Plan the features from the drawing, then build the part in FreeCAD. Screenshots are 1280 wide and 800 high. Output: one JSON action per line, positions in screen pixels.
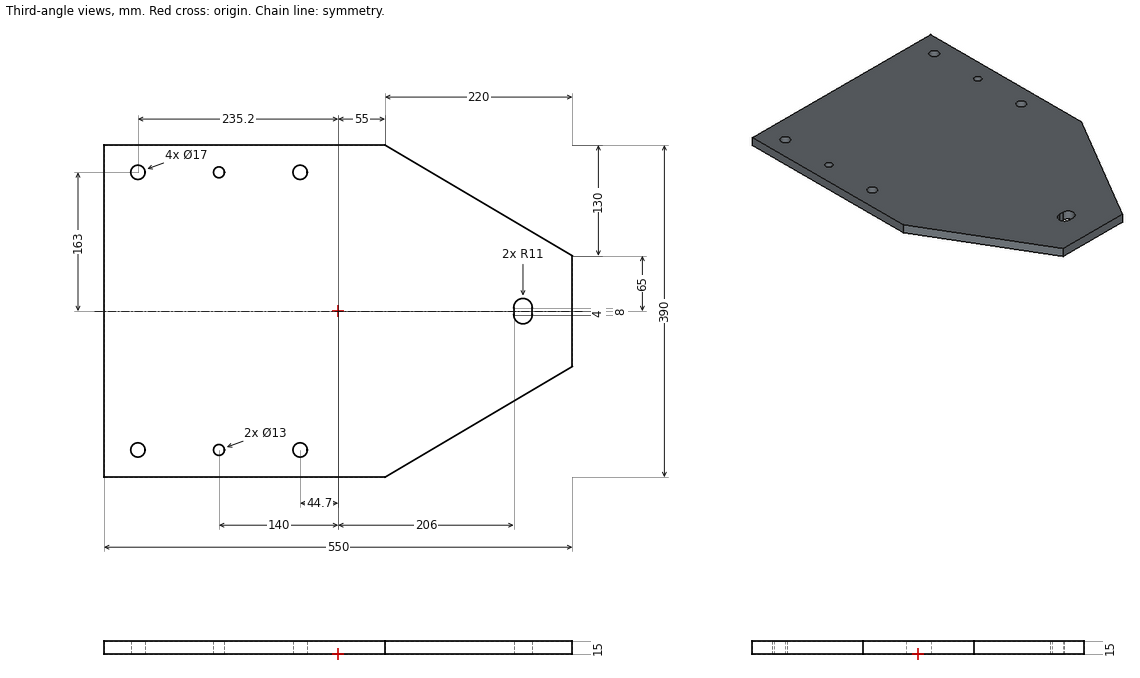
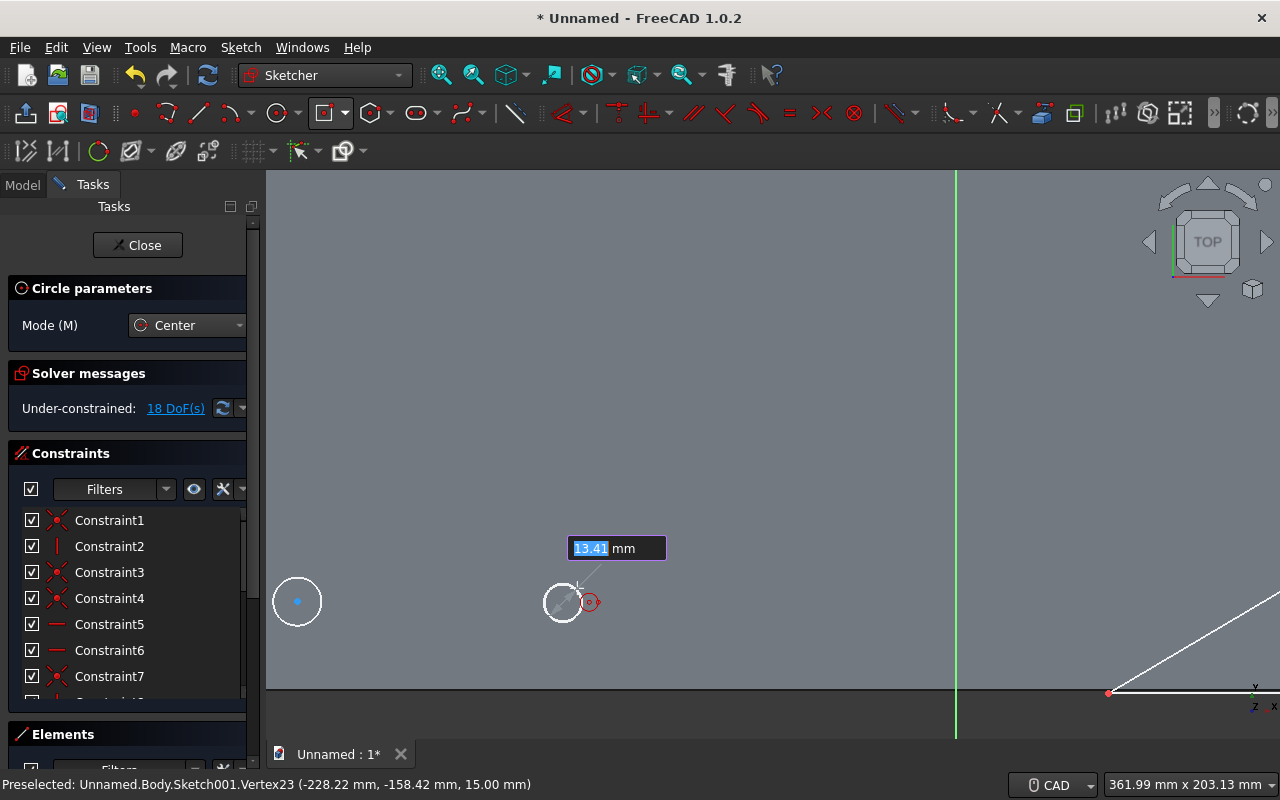
{"action": "left_click", "coordinate": [577, 587]}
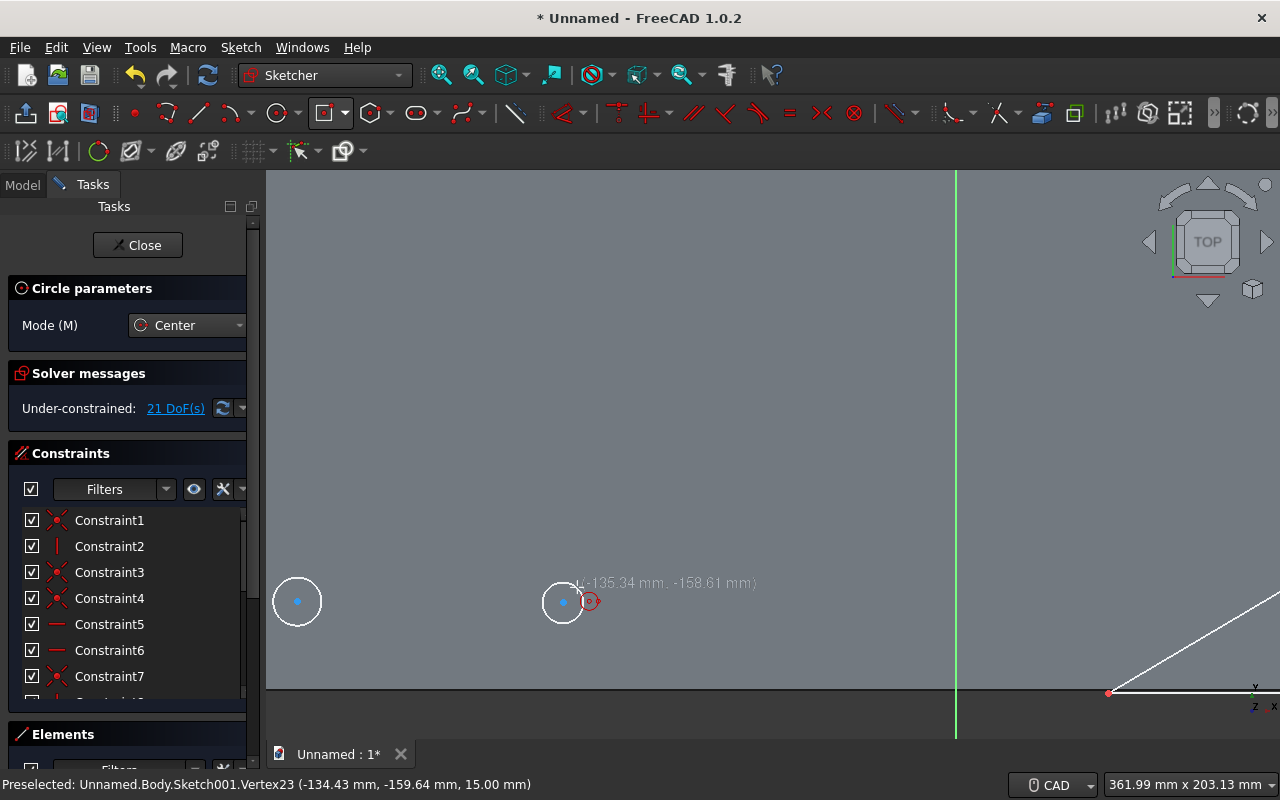
{"action": "left_click", "coordinate": [831, 600]}
{"action": "left_click", "coordinate": [848, 583]}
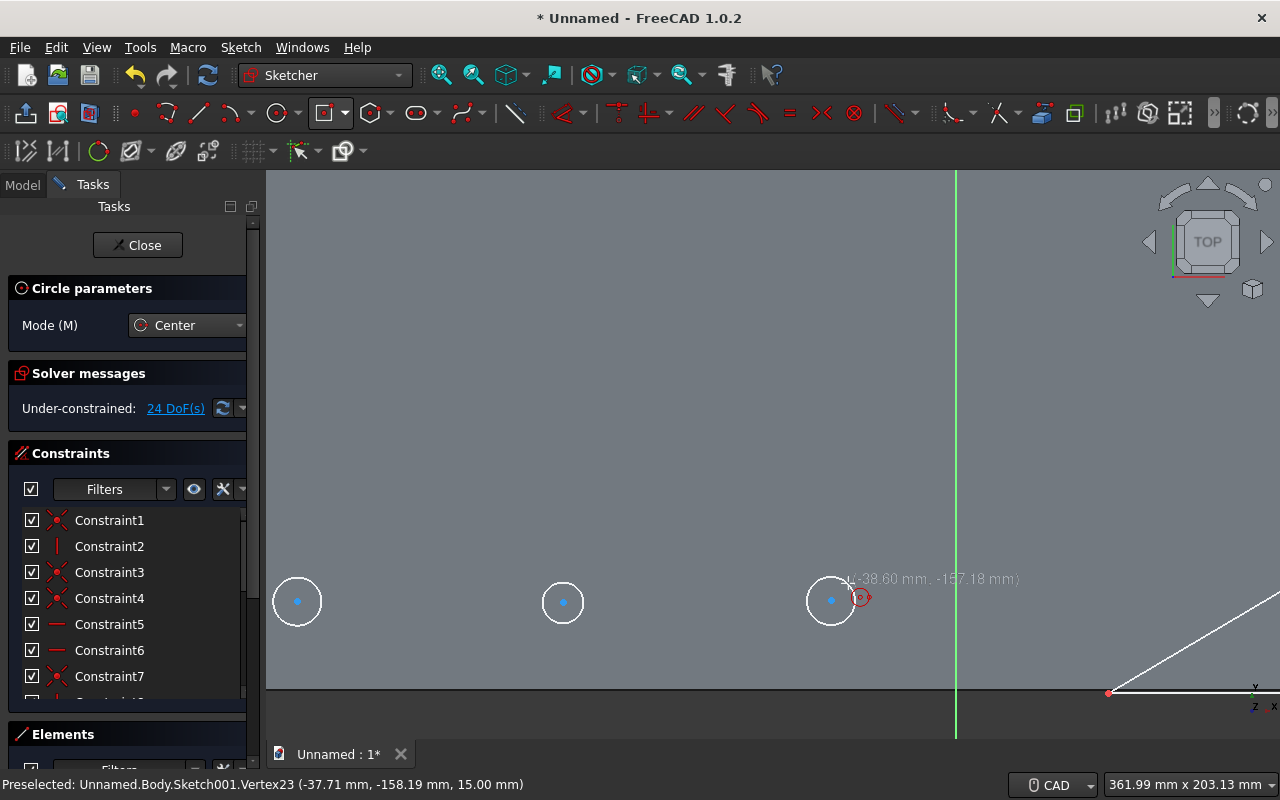
{"action": "scroll", "coordinate": [577, 588], "scroll_direction": "down", "scroll_amount": 6}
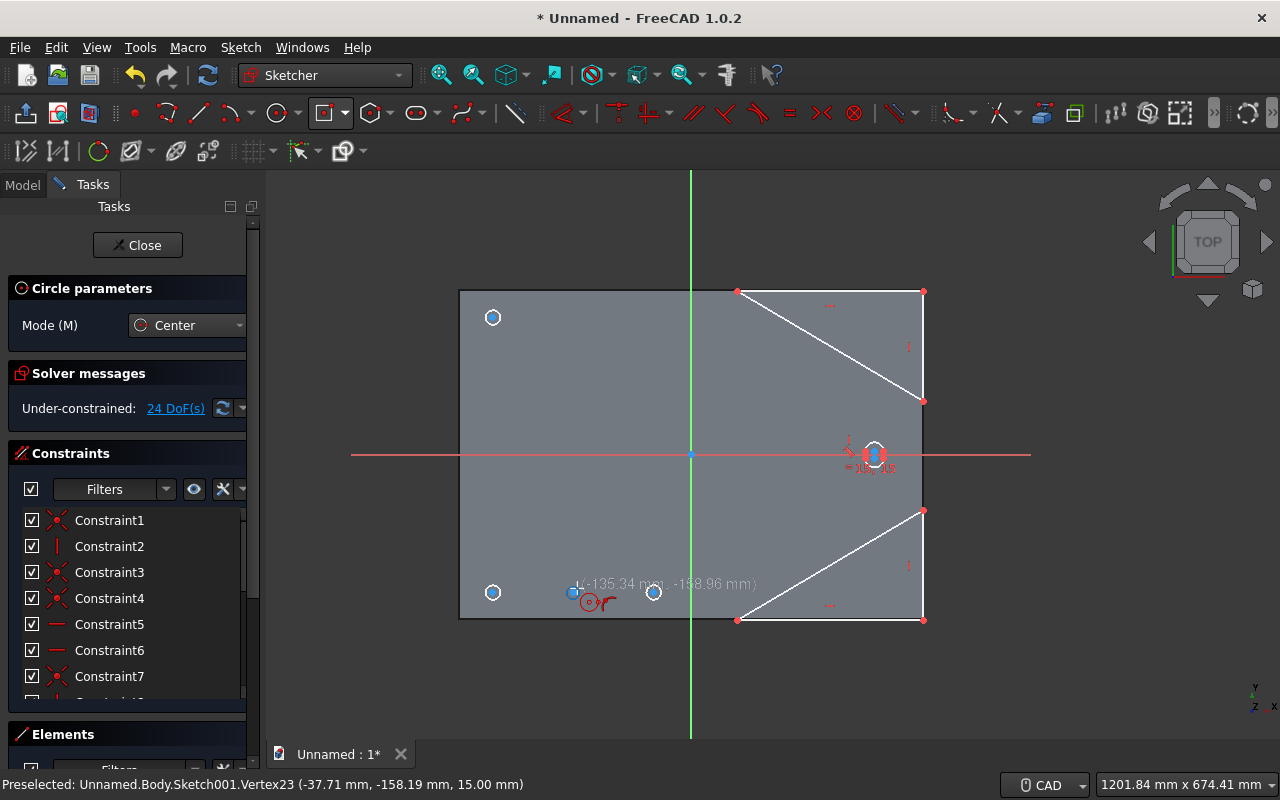
{"action": "scroll", "coordinate": [573, 317], "scroll_direction": "up", "scroll_amount": 8}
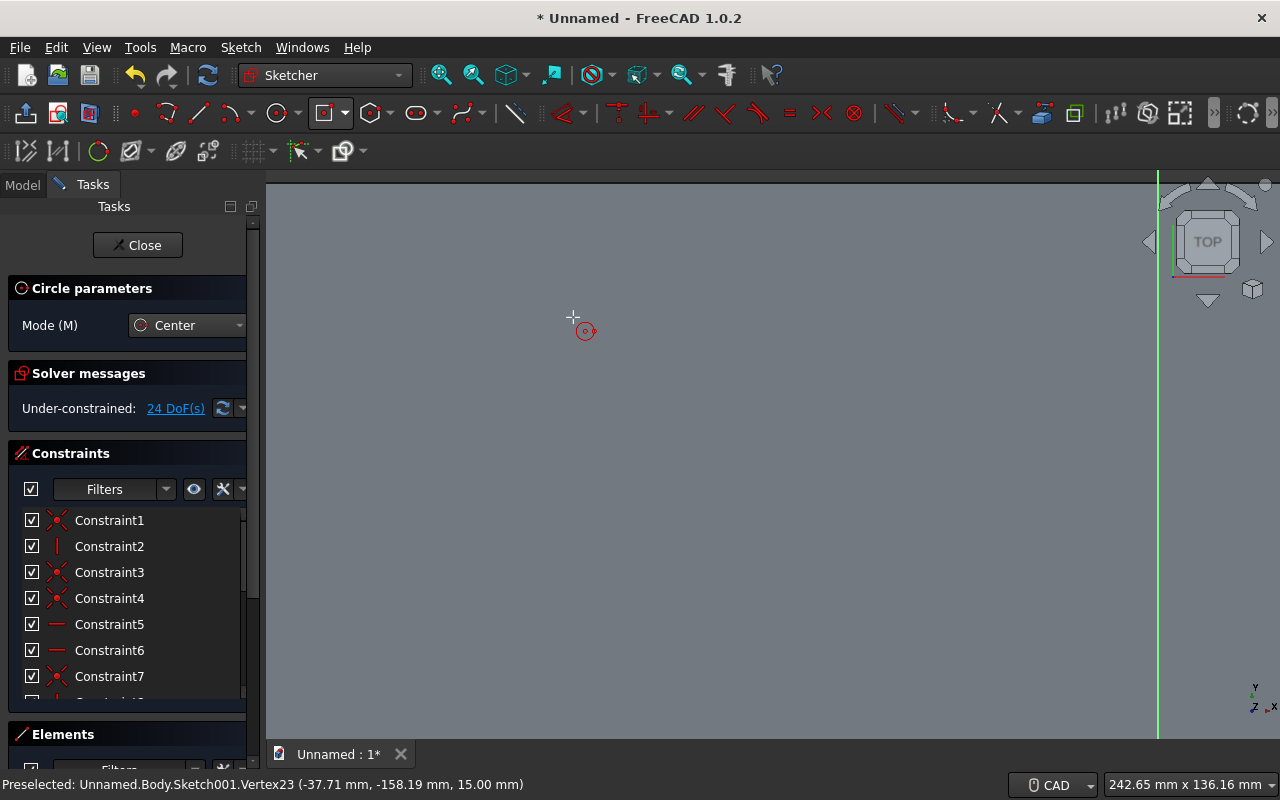
{"action": "scroll", "coordinate": [573, 317], "scroll_direction": "down", "scroll_amount": 8}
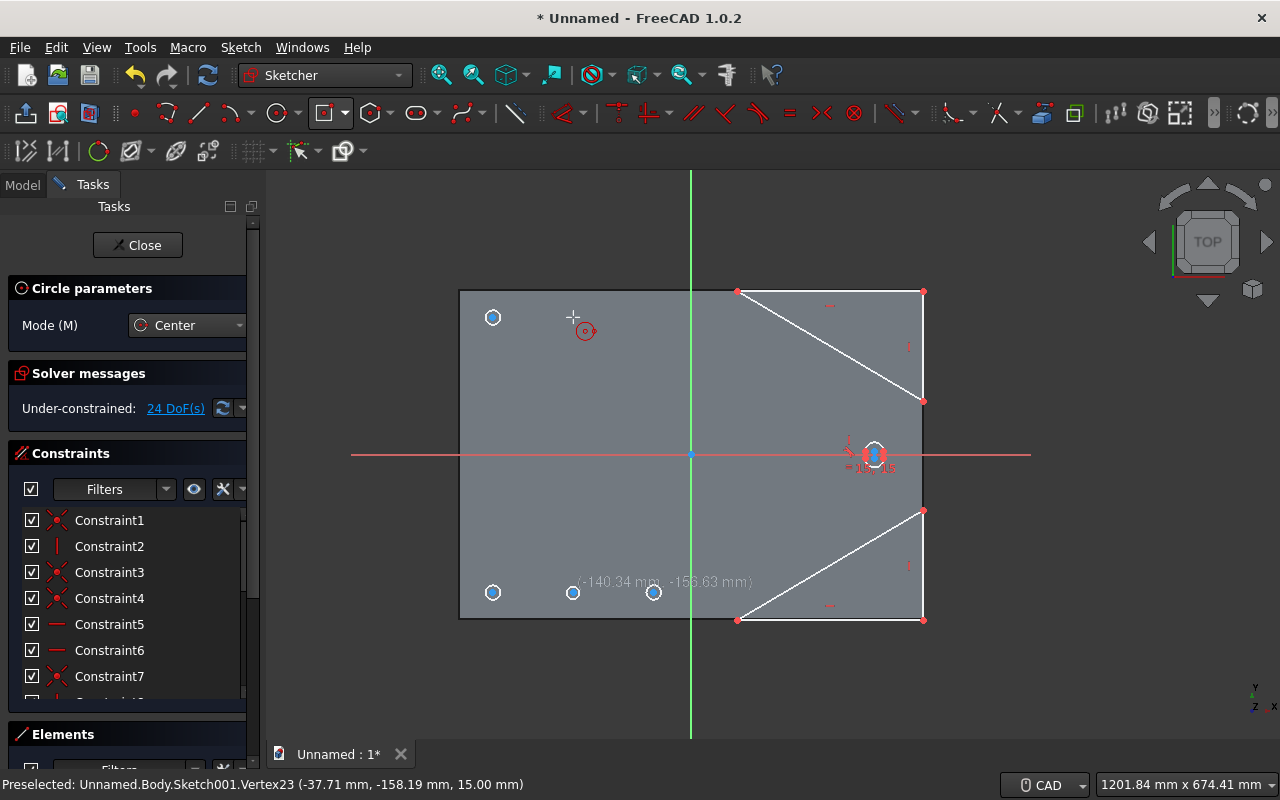
{"action": "left_click", "coordinate": [573, 317]}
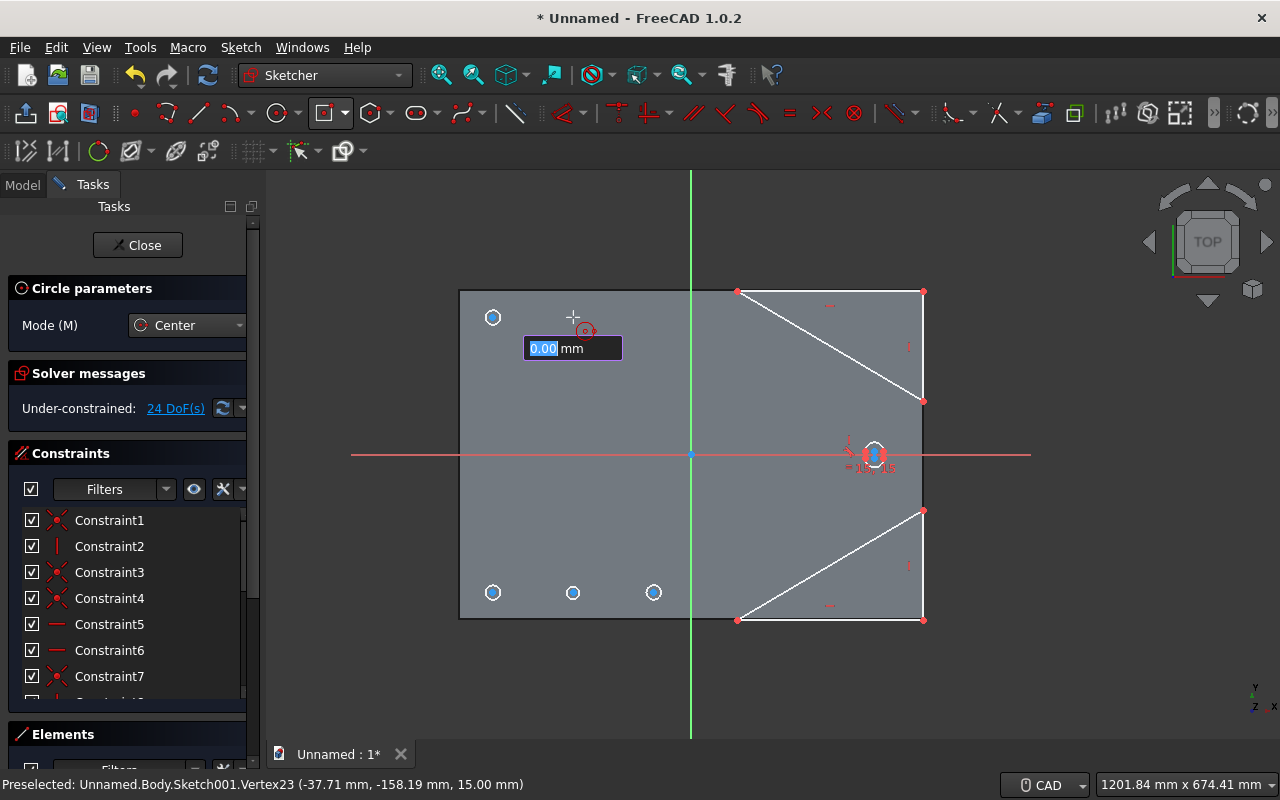
{"action": "scroll", "coordinate": [577, 313], "scroll_direction": "up", "scroll_amount": 6}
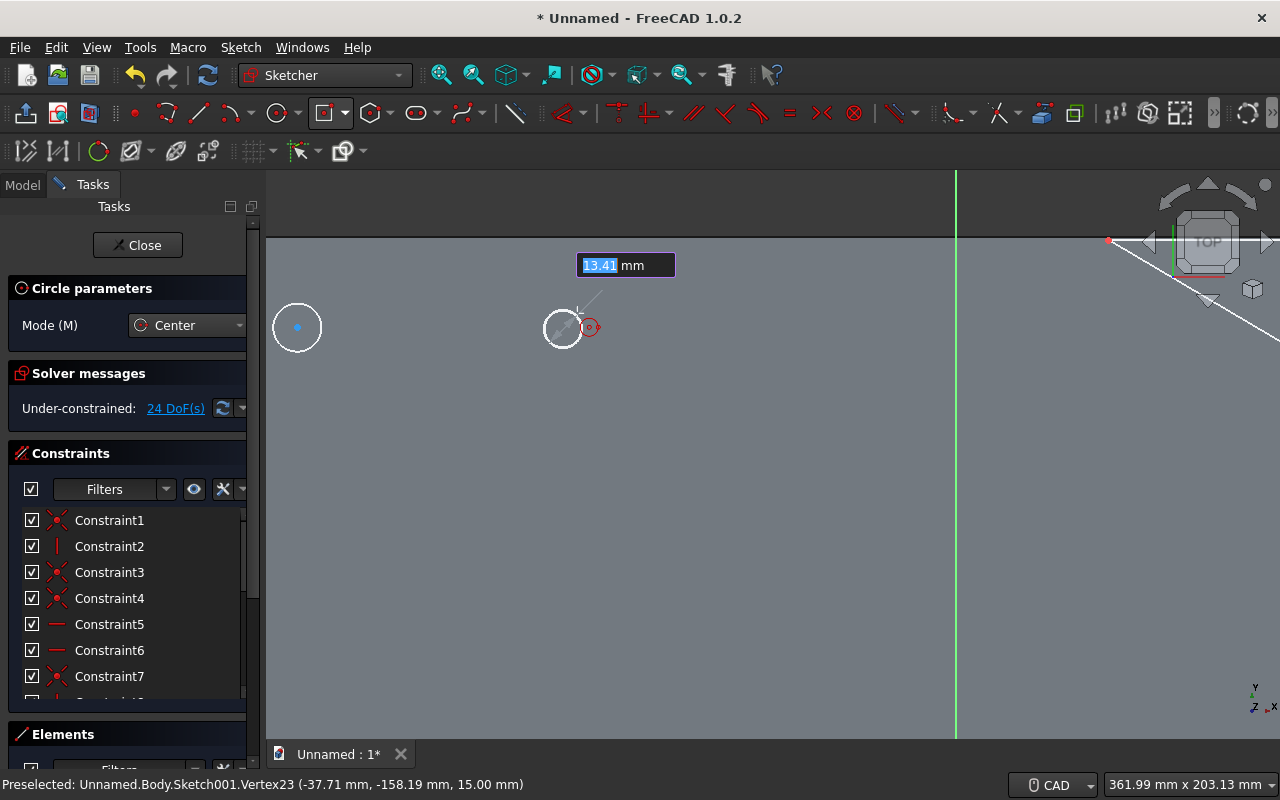
{"action": "left_click", "coordinate": [577, 313]}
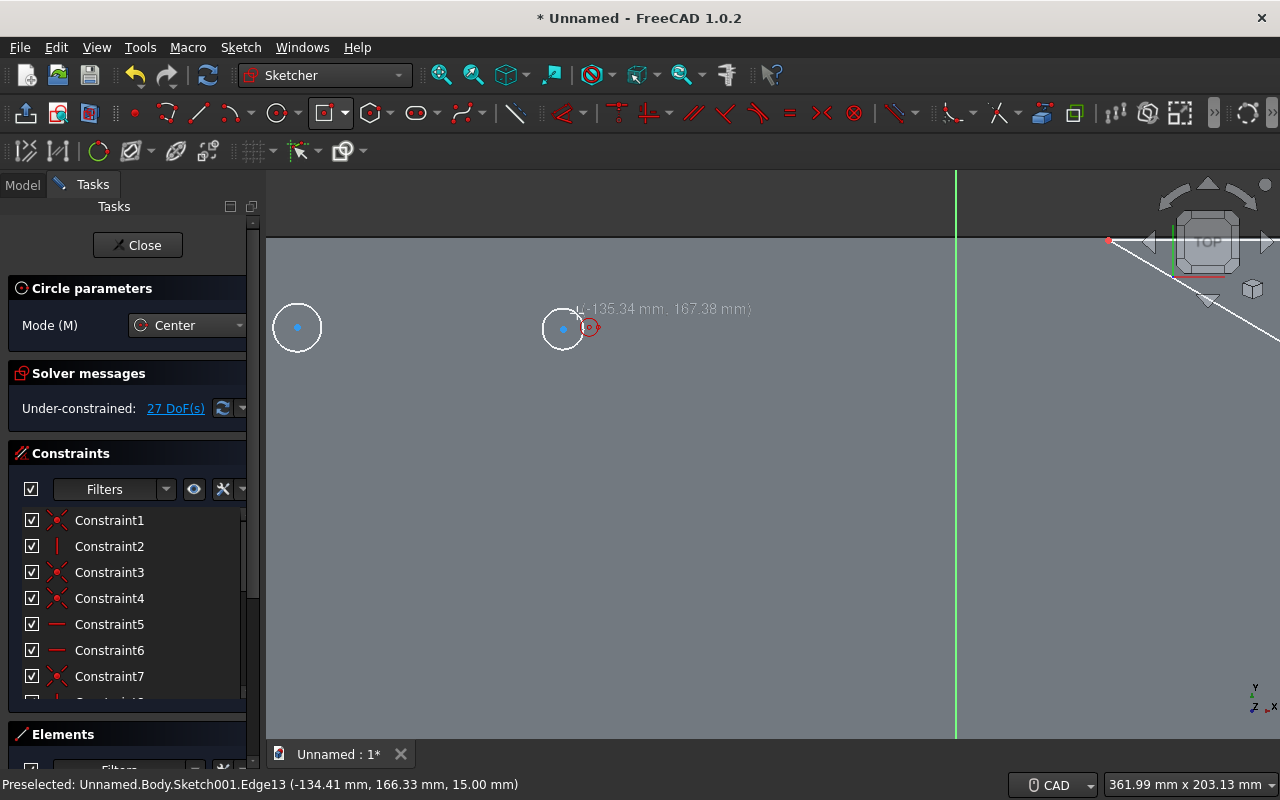
{"action": "left_click", "coordinate": [831, 326]}
{"action": "left_click", "coordinate": [848, 309]}
{"action": "key", "text": "Escape"}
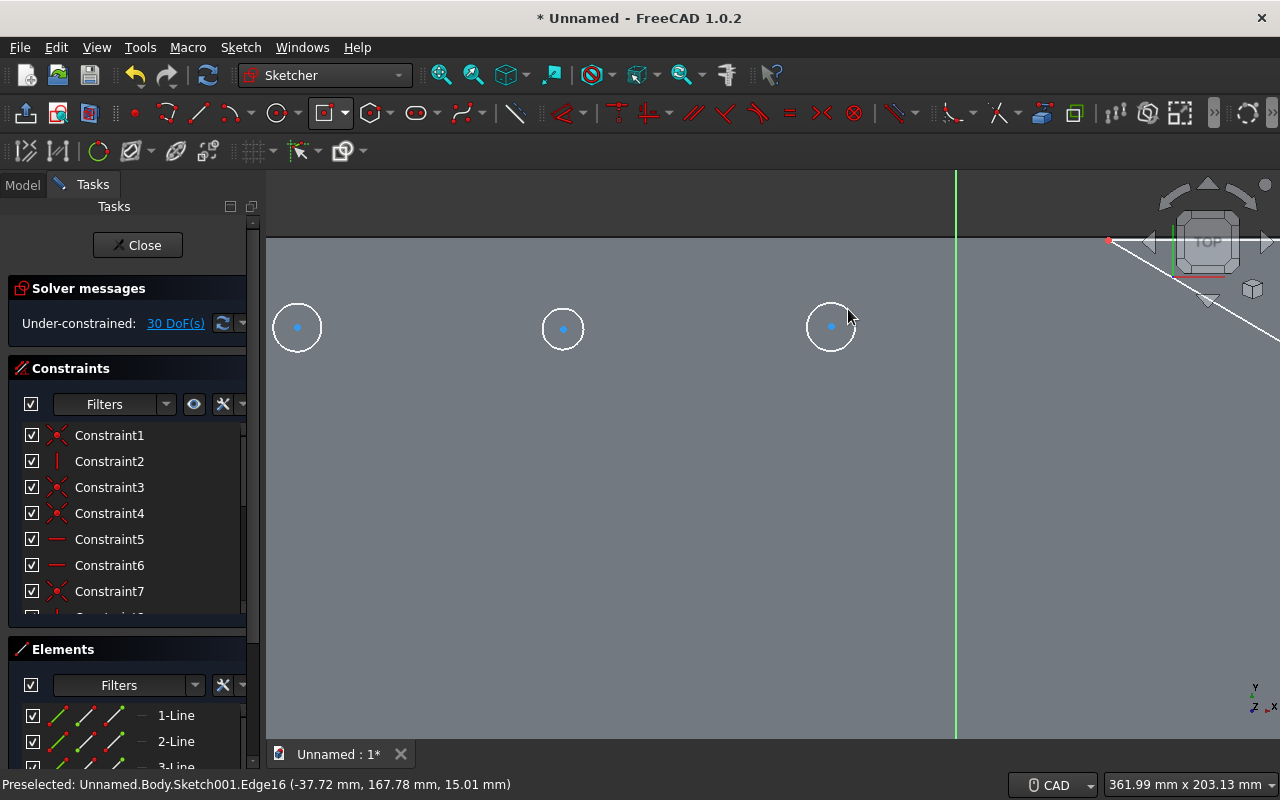
{"action": "left_click", "coordinate": [314, 311]}